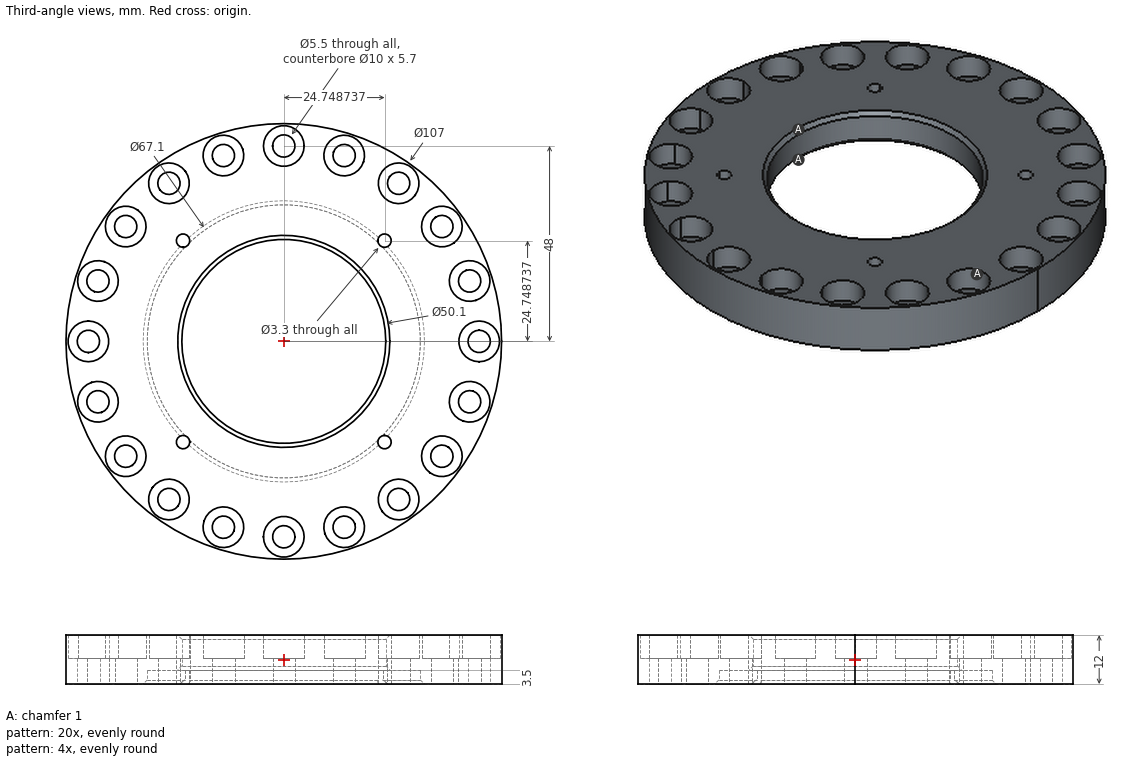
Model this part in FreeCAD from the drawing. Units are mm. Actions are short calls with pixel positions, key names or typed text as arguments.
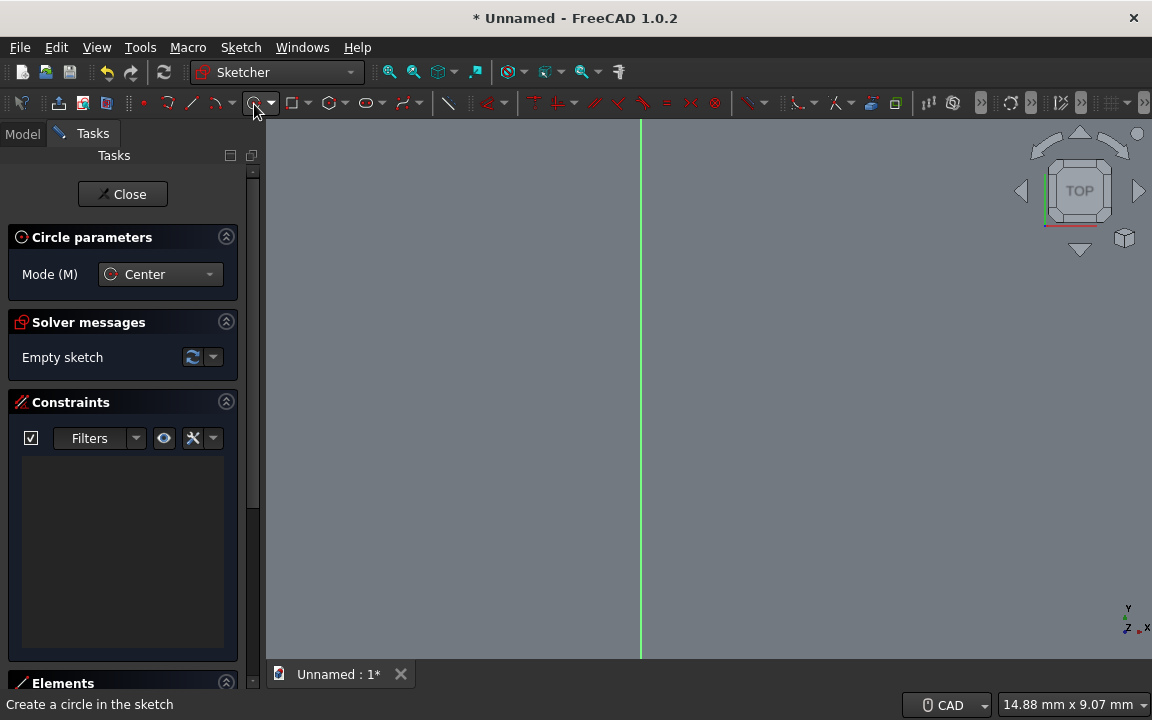
click(641, 389)
click(756, 273)
key(Escape)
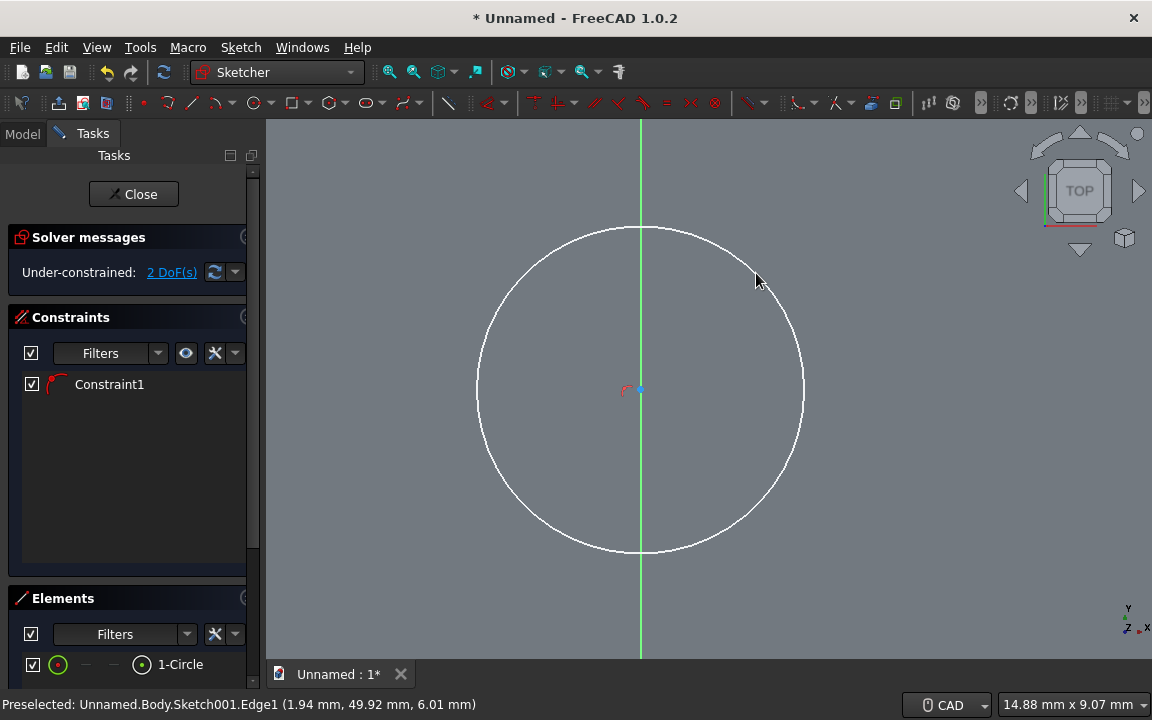
click(488, 104)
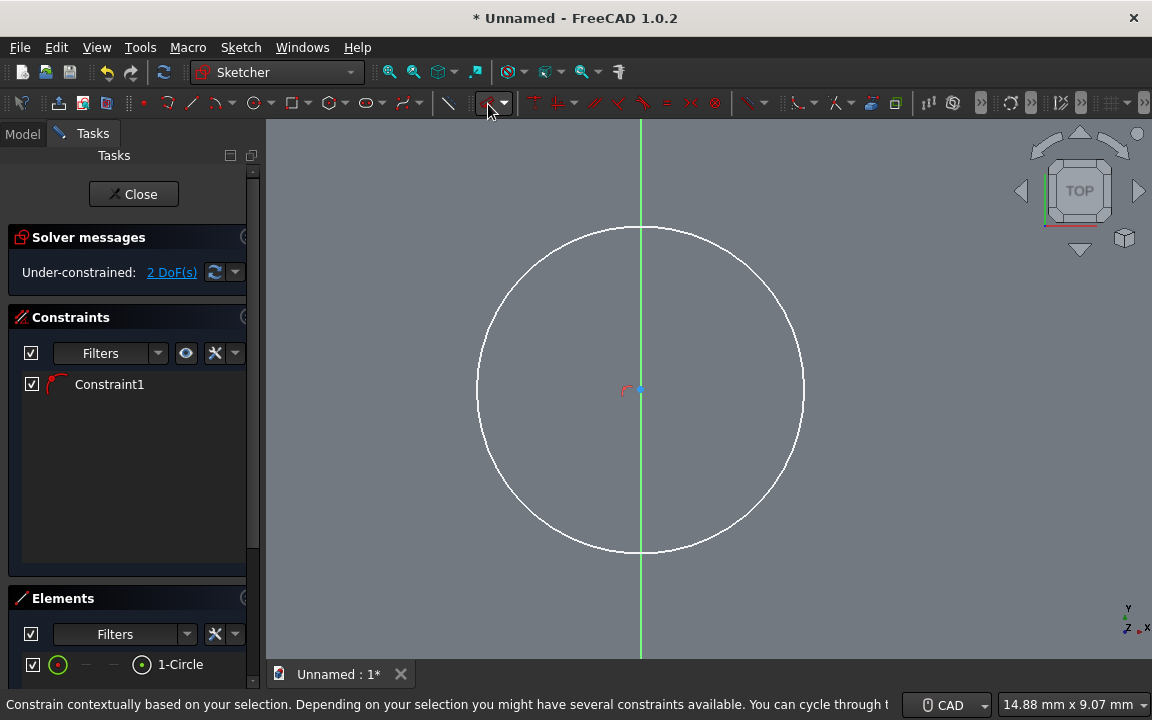
click(756, 274)
click(779, 251)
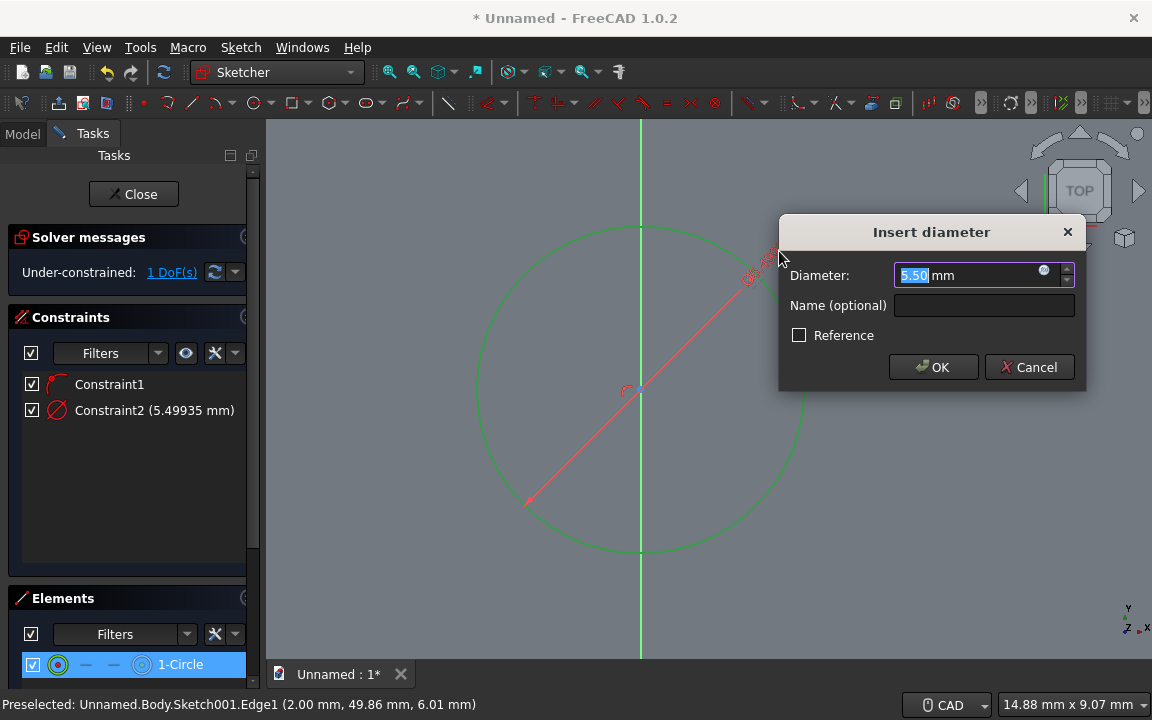
text(5.5)
key(Return)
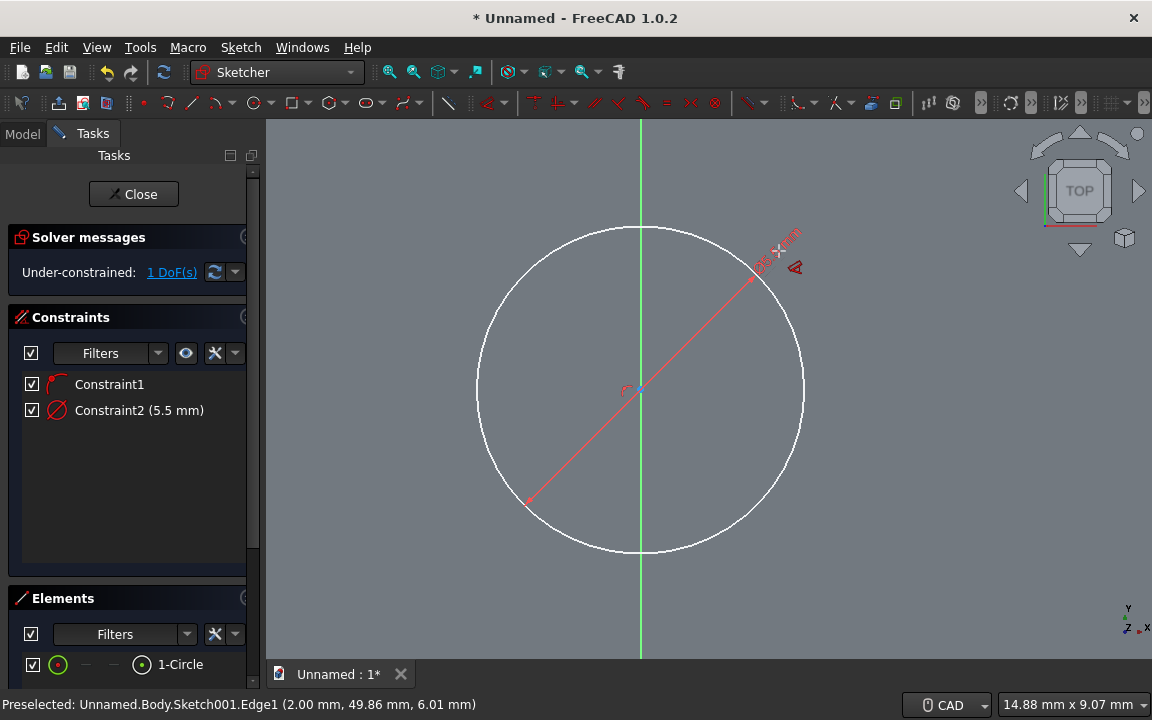
click(641, 390)
click(675, 510)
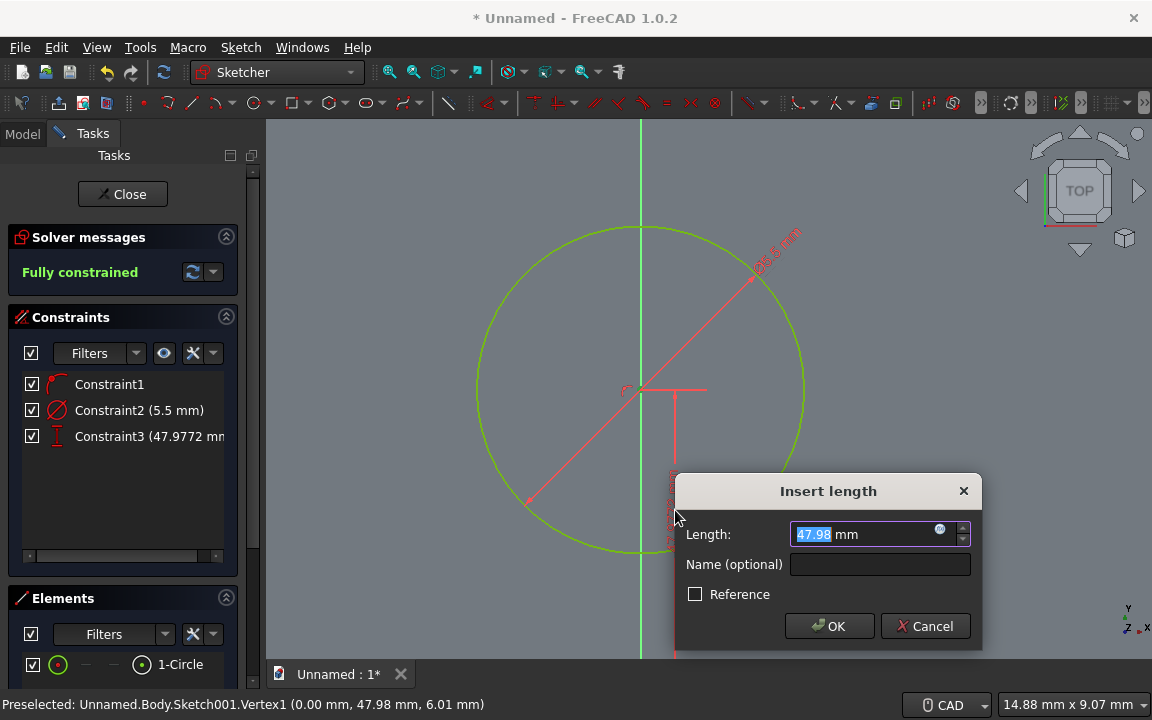
text(48)
key(Return)
key(Escape)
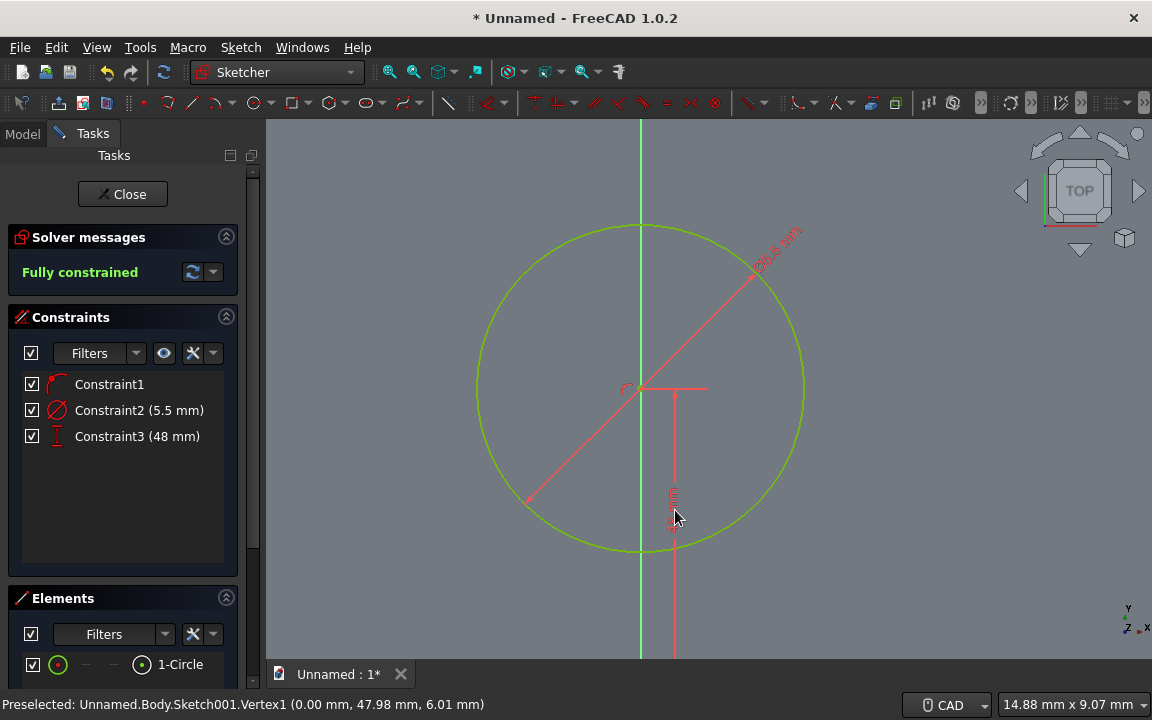
click(123, 194)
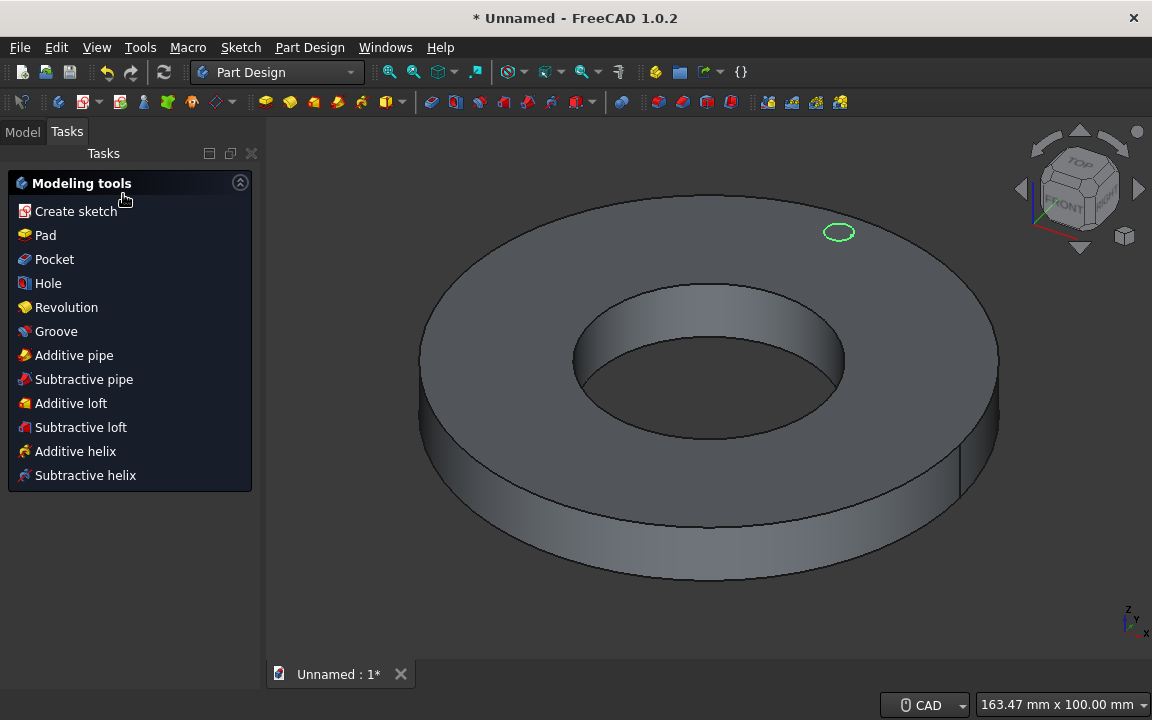
click(456, 102)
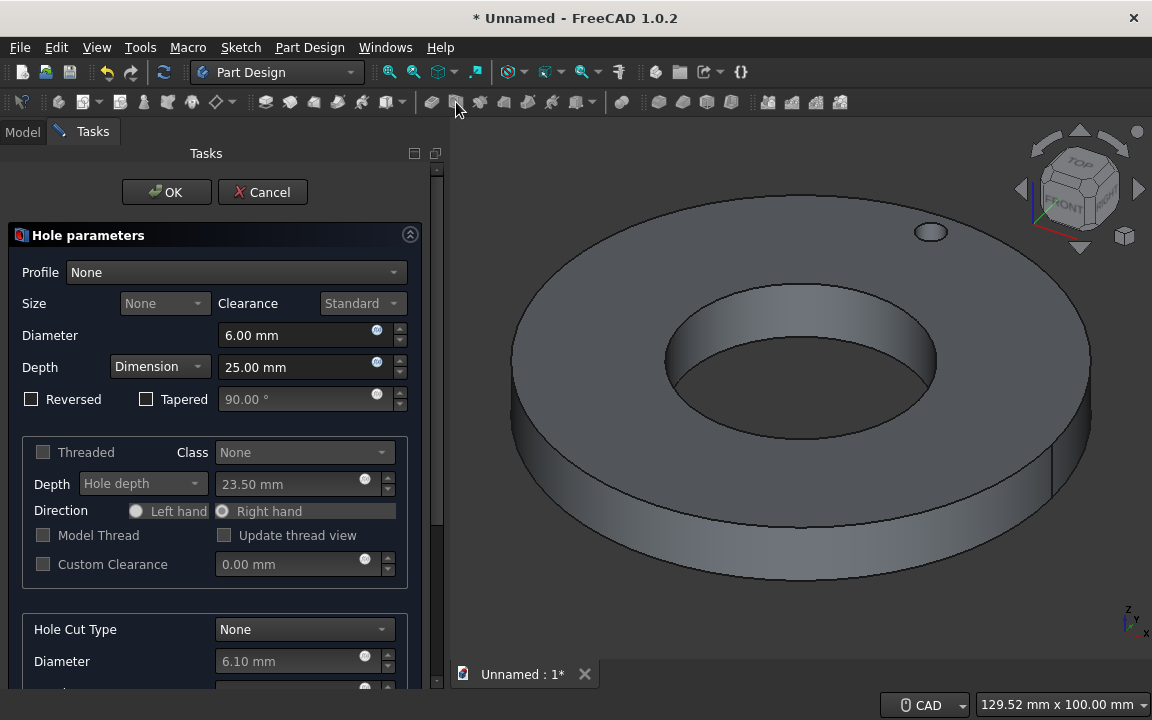
triple_click(305, 335)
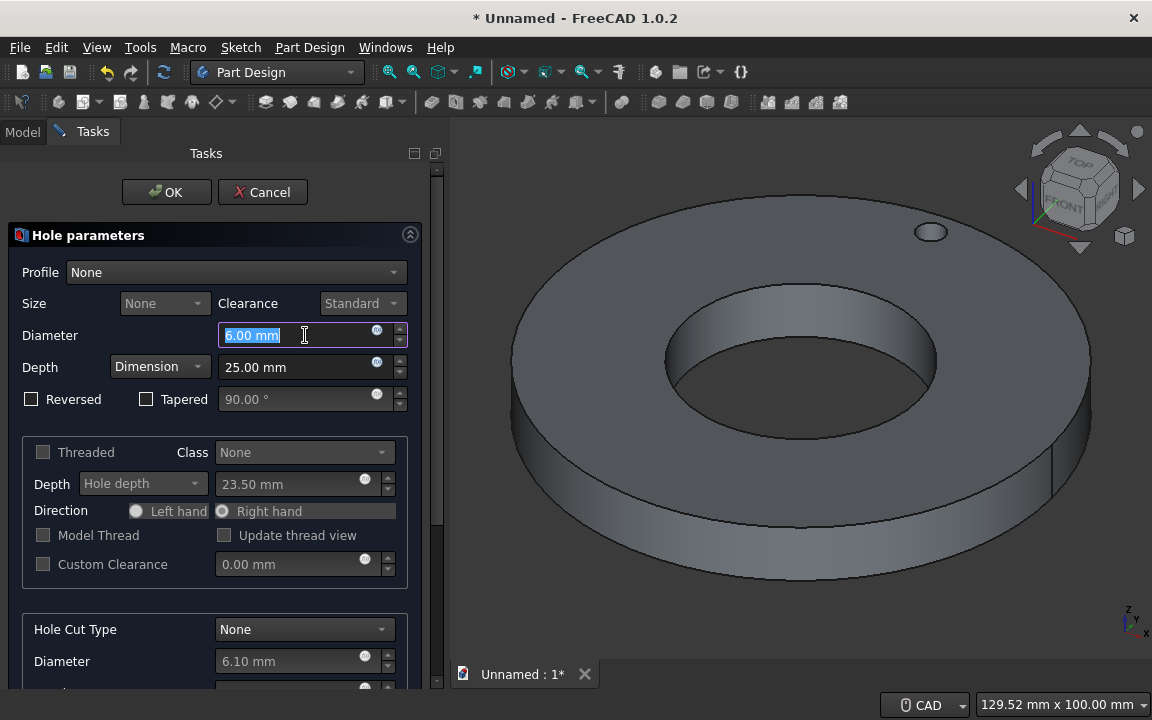
text(5.5)
key(Tab)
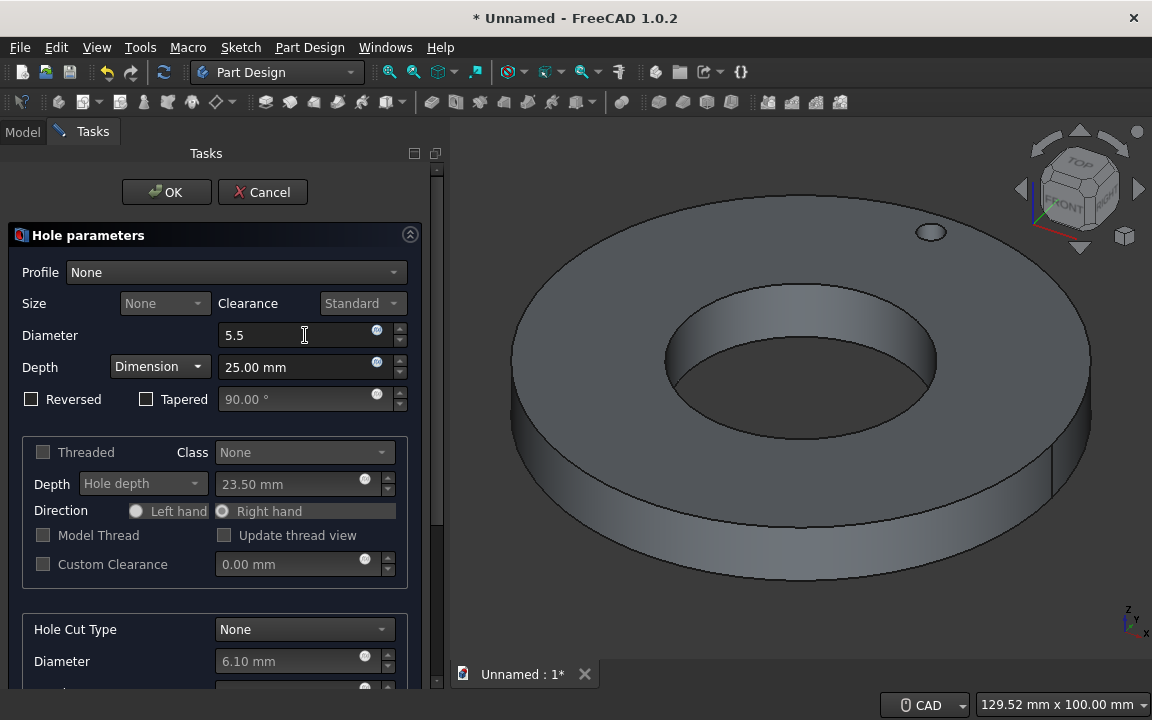
click(161, 366)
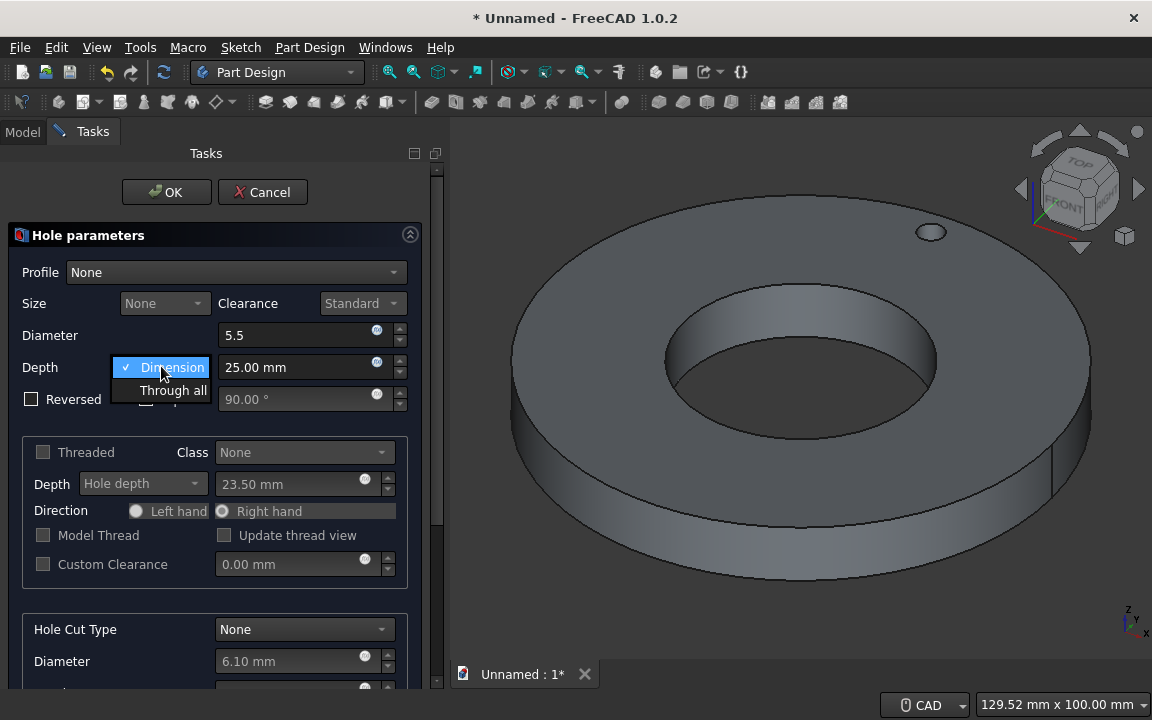
click(160, 390)